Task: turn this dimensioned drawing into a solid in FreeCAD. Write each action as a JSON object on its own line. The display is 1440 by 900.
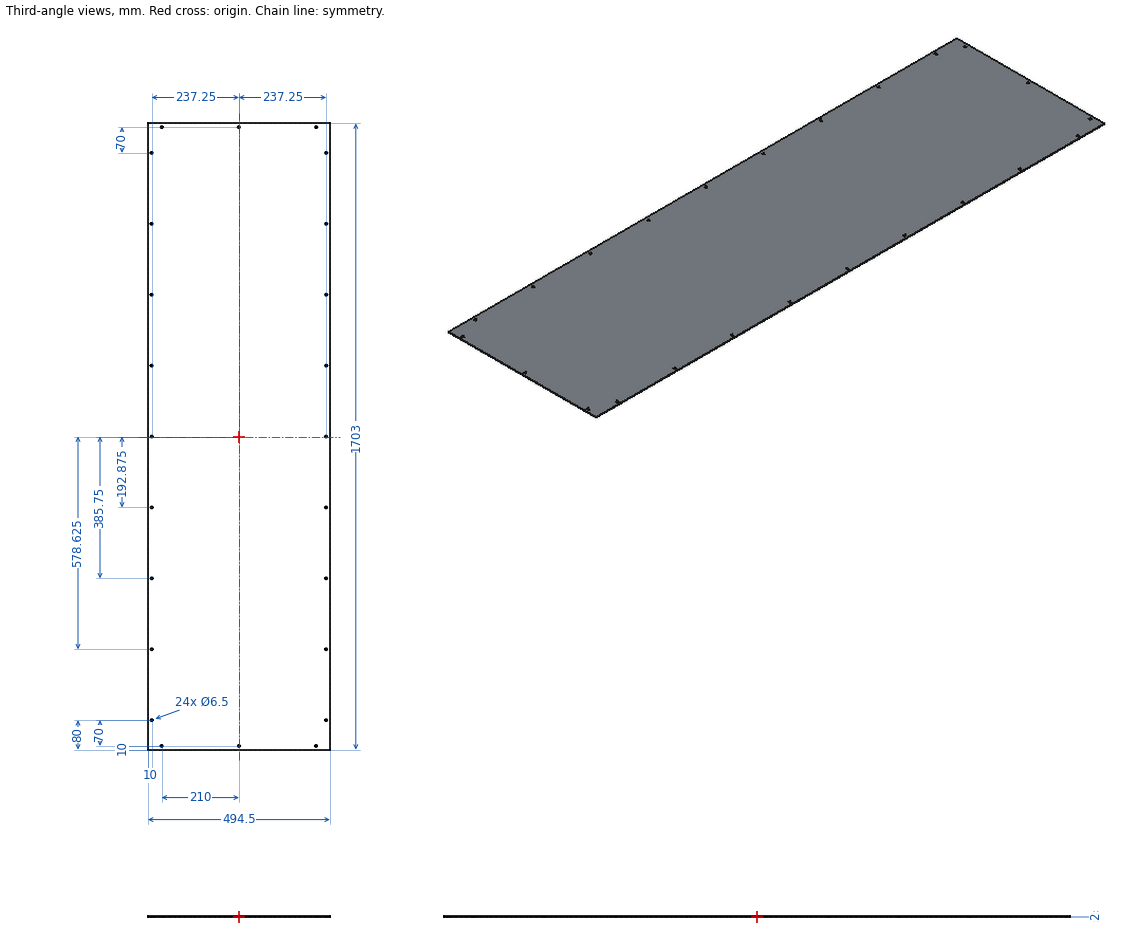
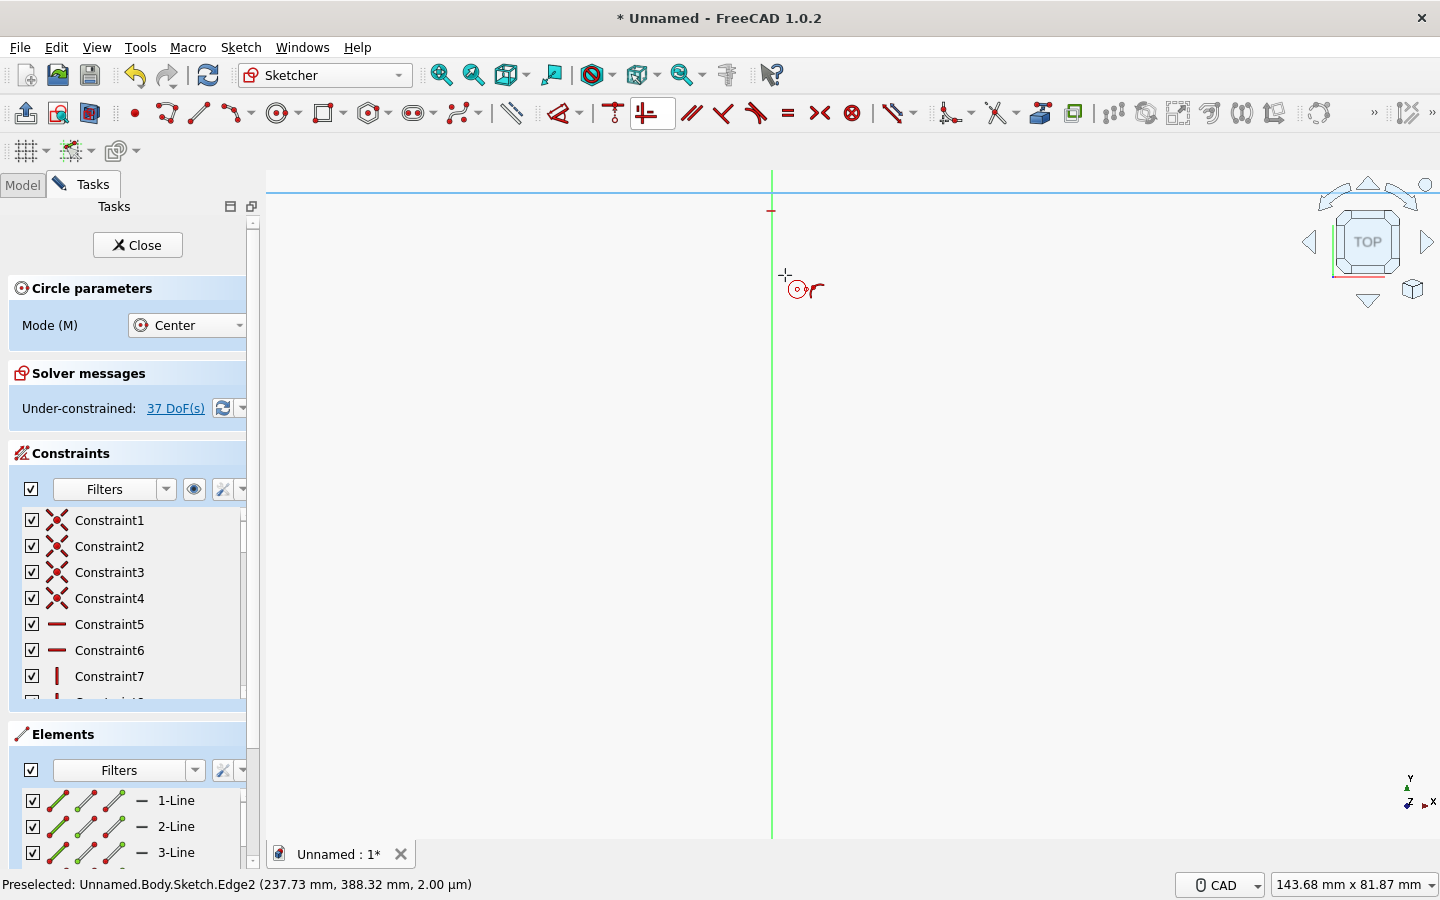
{"action": "scroll", "coordinate": [785, 275], "scroll_direction": "down", "scroll_amount": 17}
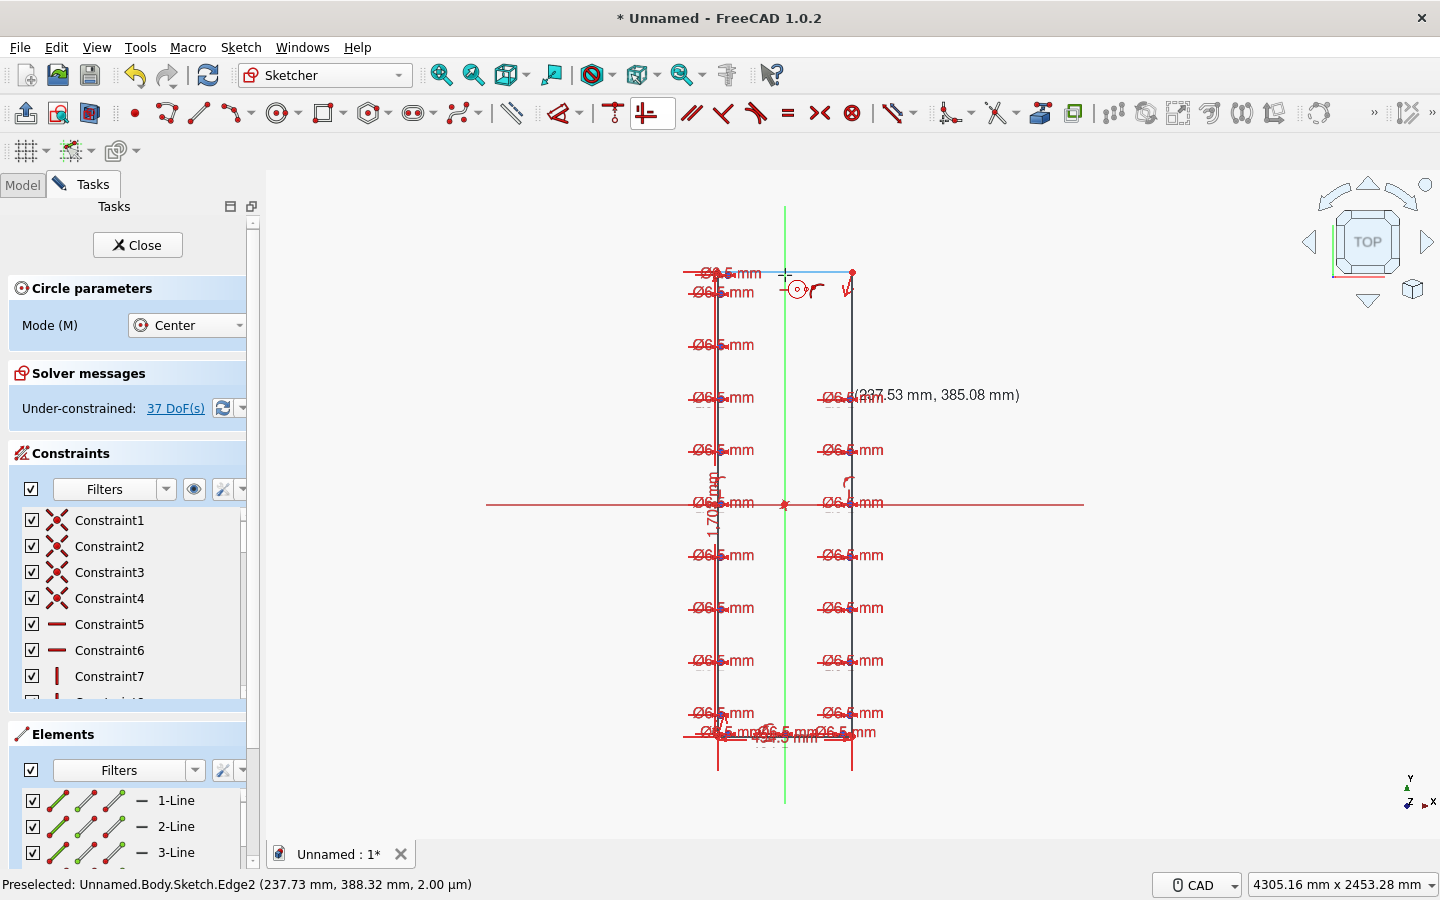
{"action": "scroll", "coordinate": [785, 275], "scroll_direction": "up", "scroll_amount": 9}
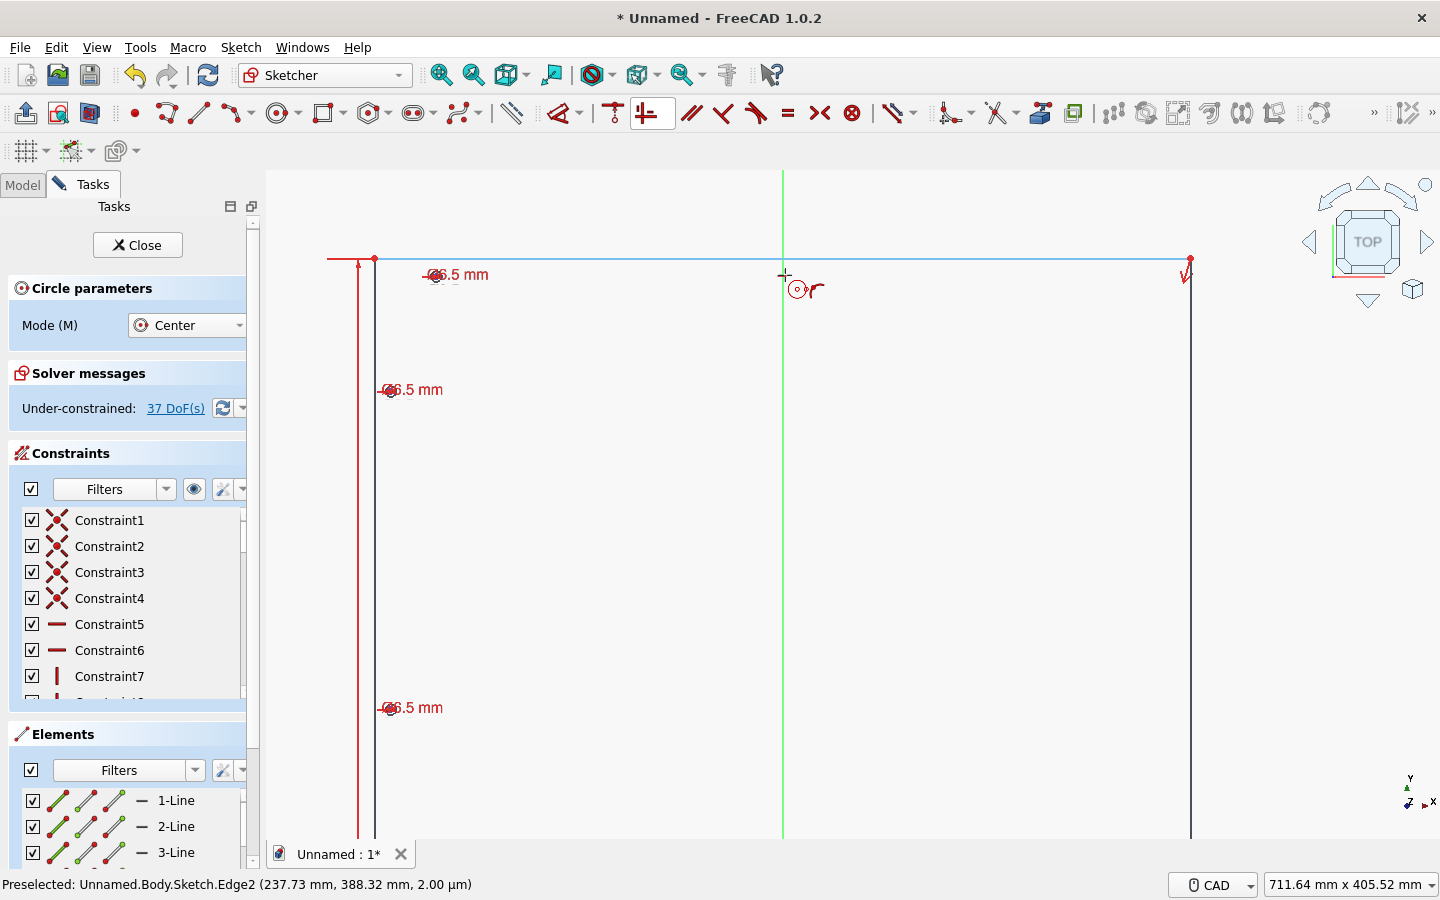
{"action": "left_click", "coordinate": [783, 275]}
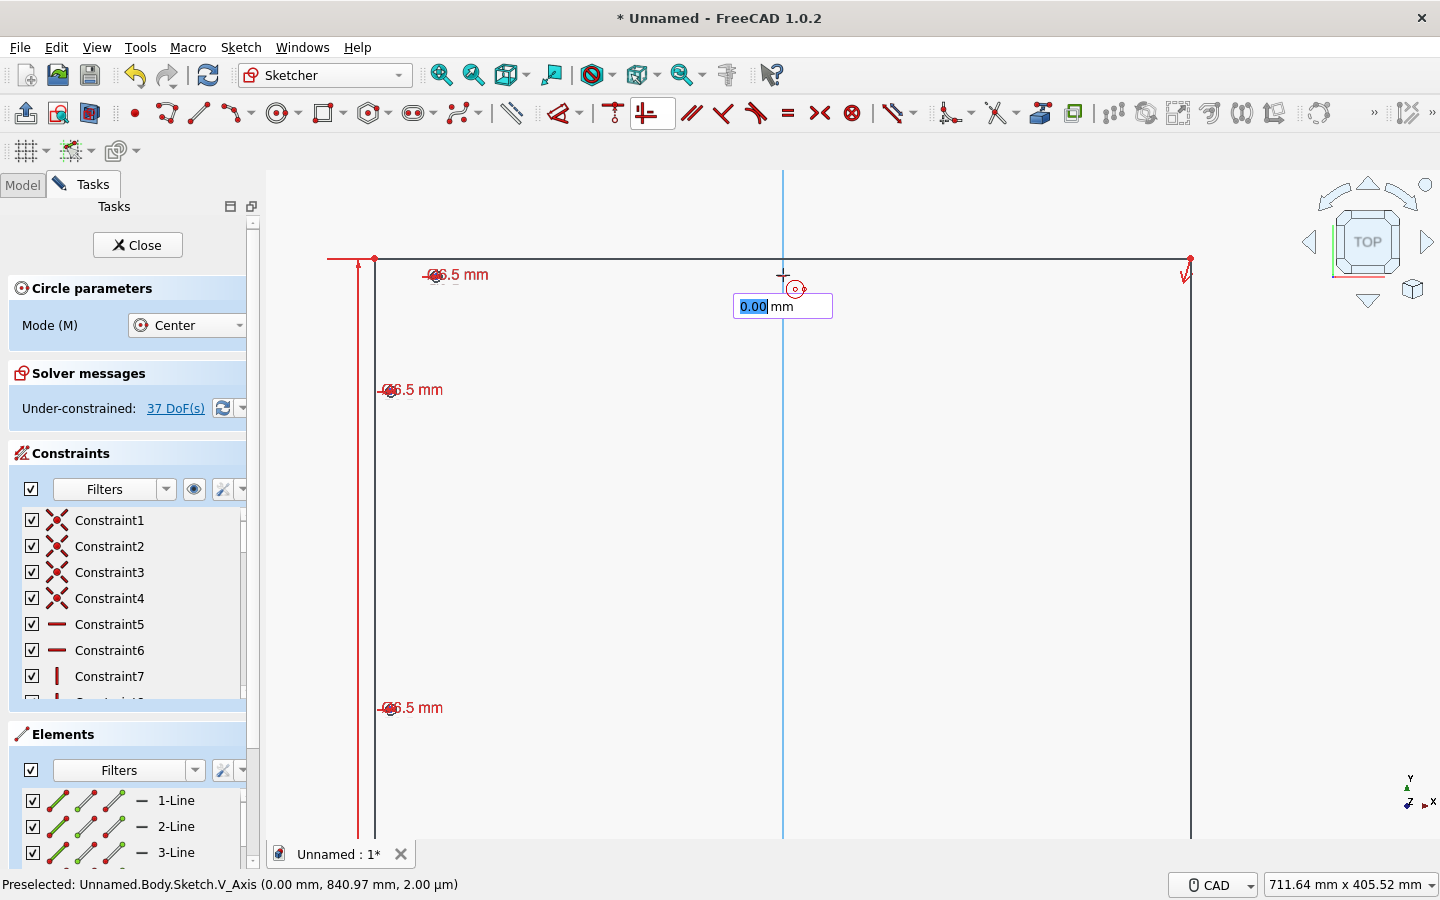
{"action": "scroll", "coordinate": [788, 273], "scroll_direction": "up", "scroll_amount": 6}
{"action": "mouse_move", "coordinate": [786, 274]}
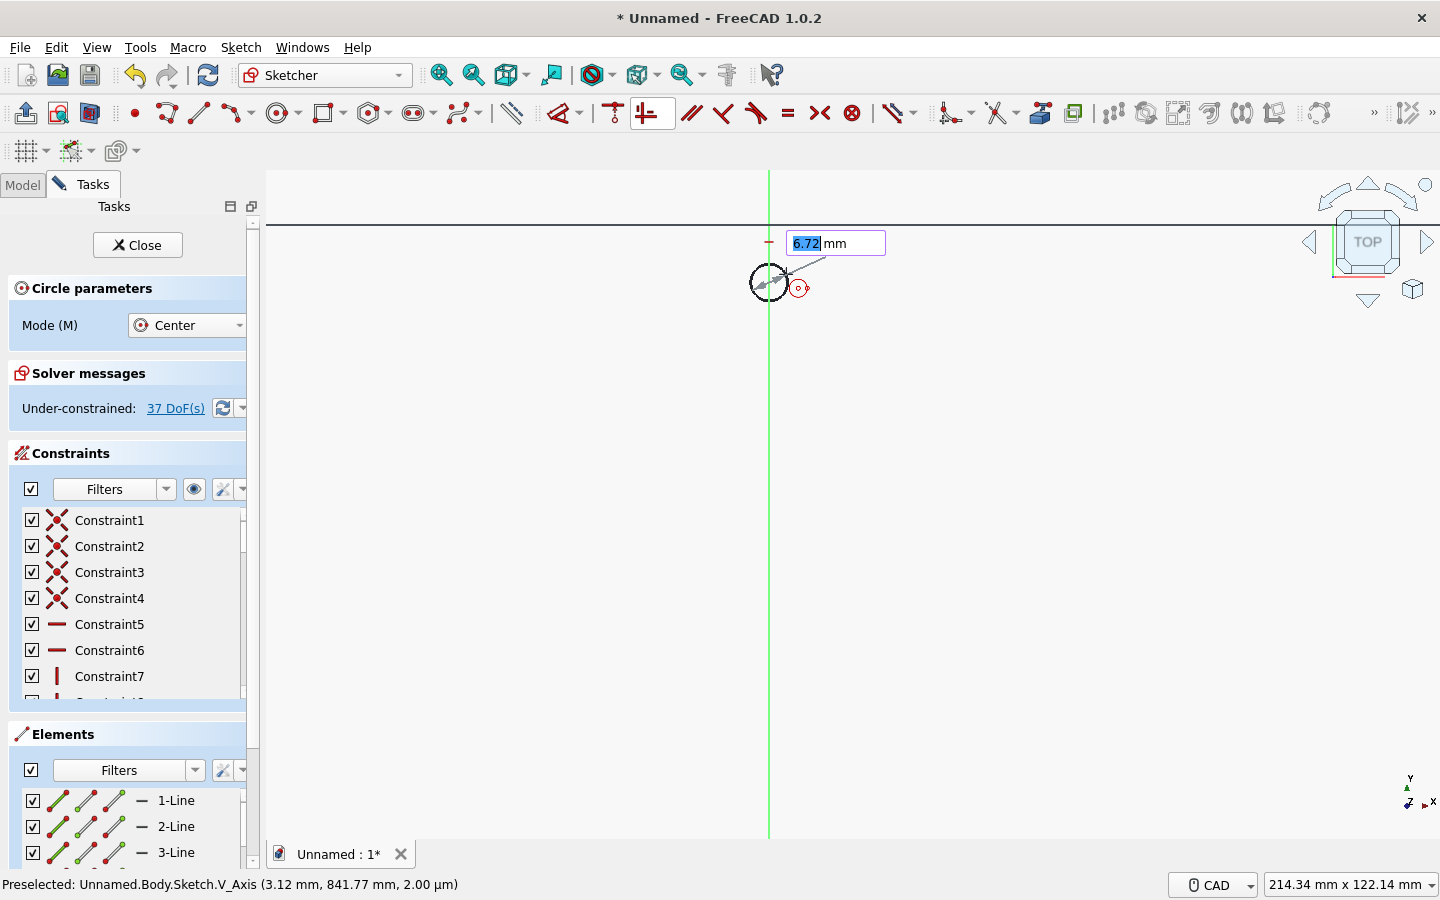
{"action": "type", "text": "6.5"}
{"action": "key", "text": "Return"}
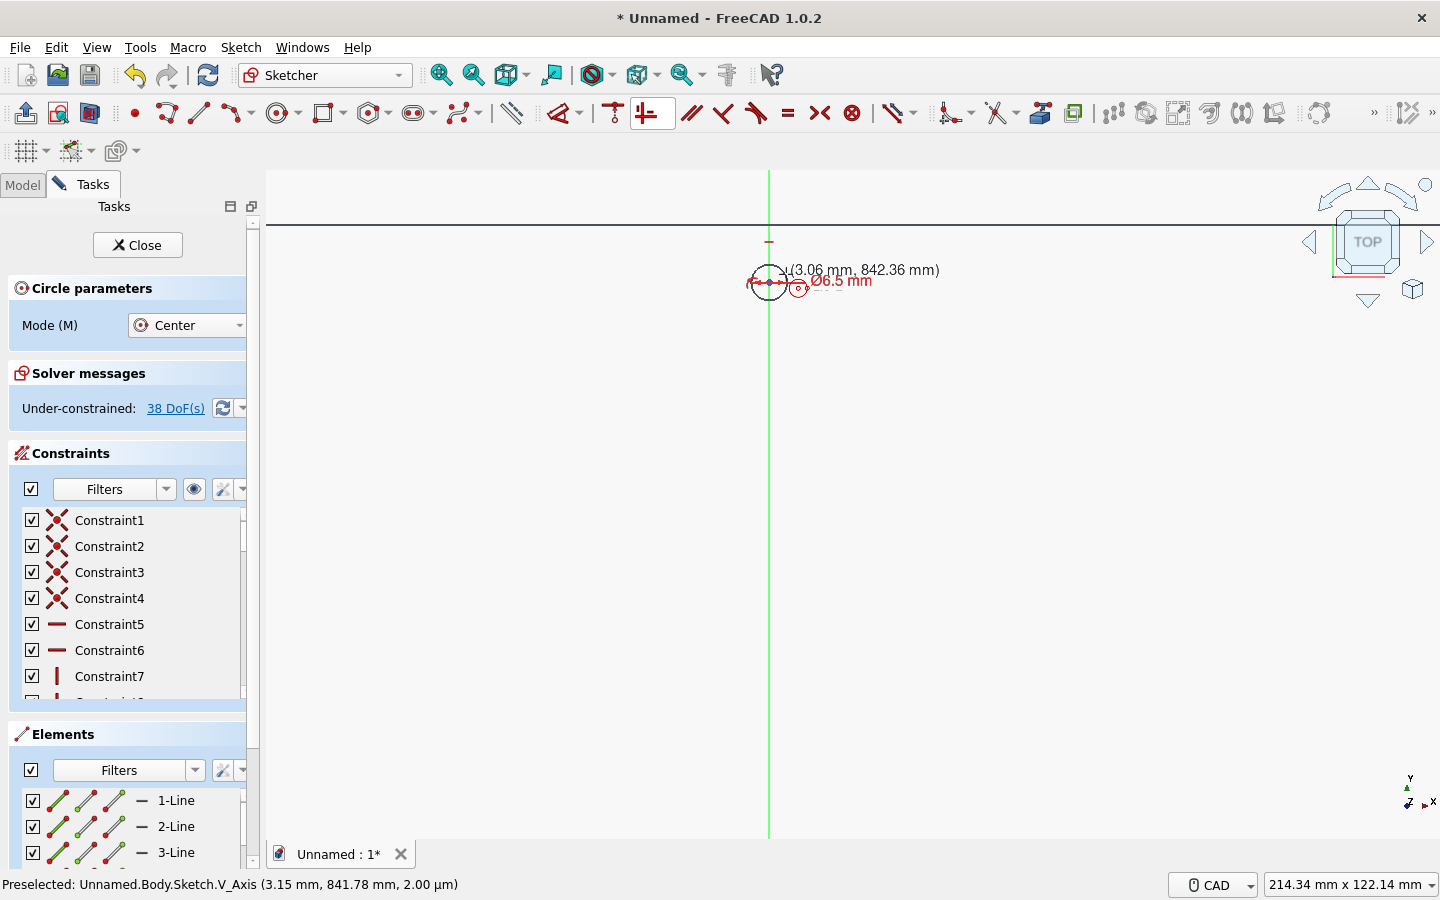
{"action": "scroll", "coordinate": [785, 275], "scroll_direction": "down", "scroll_amount": 15}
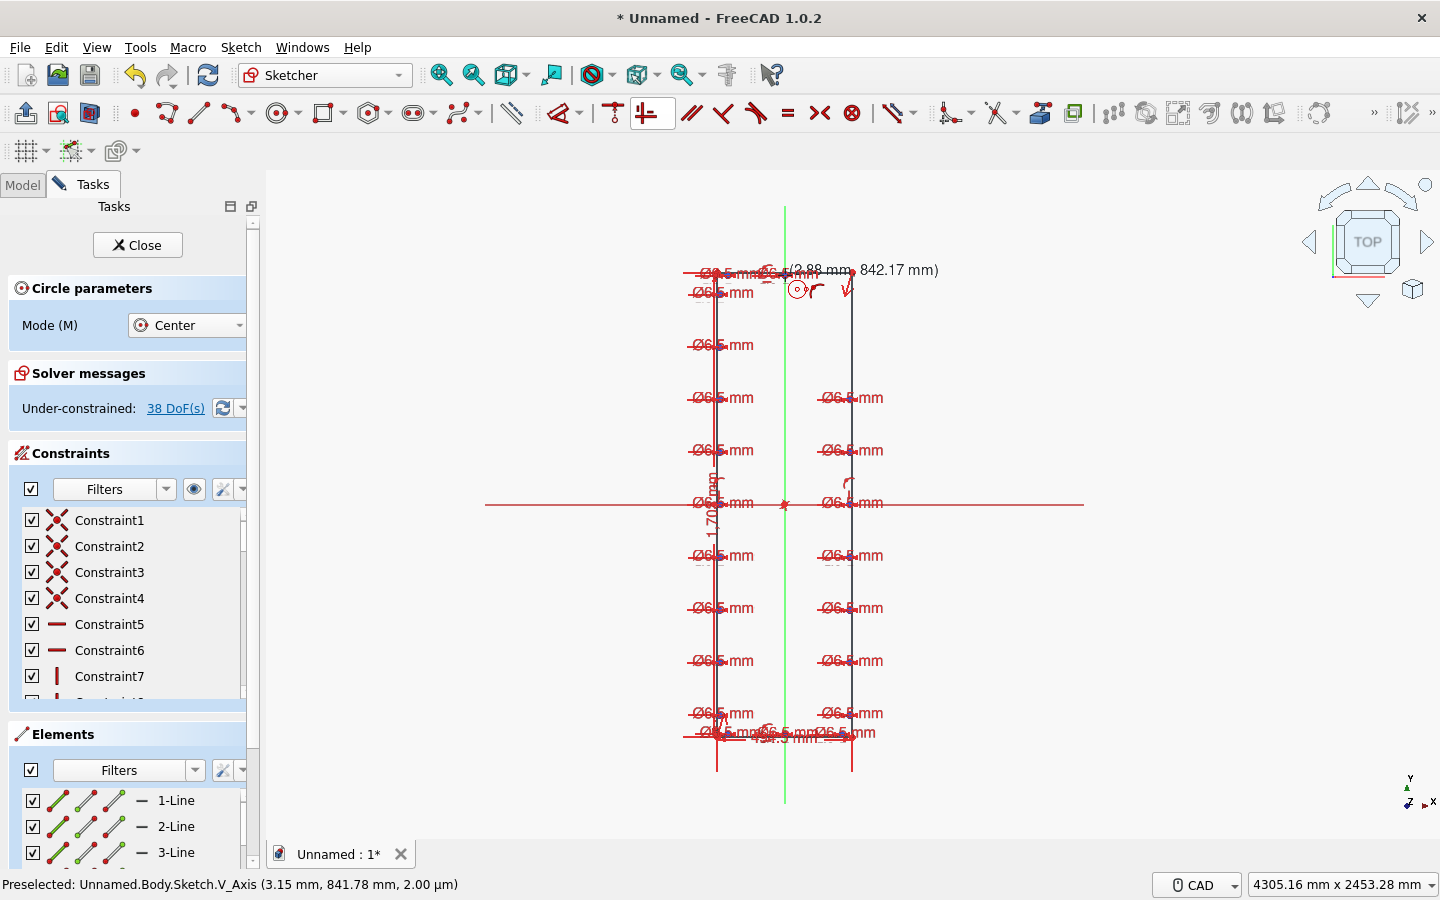
{"action": "scroll", "coordinate": [849, 347], "scroll_direction": "up", "scroll_amount": 17}